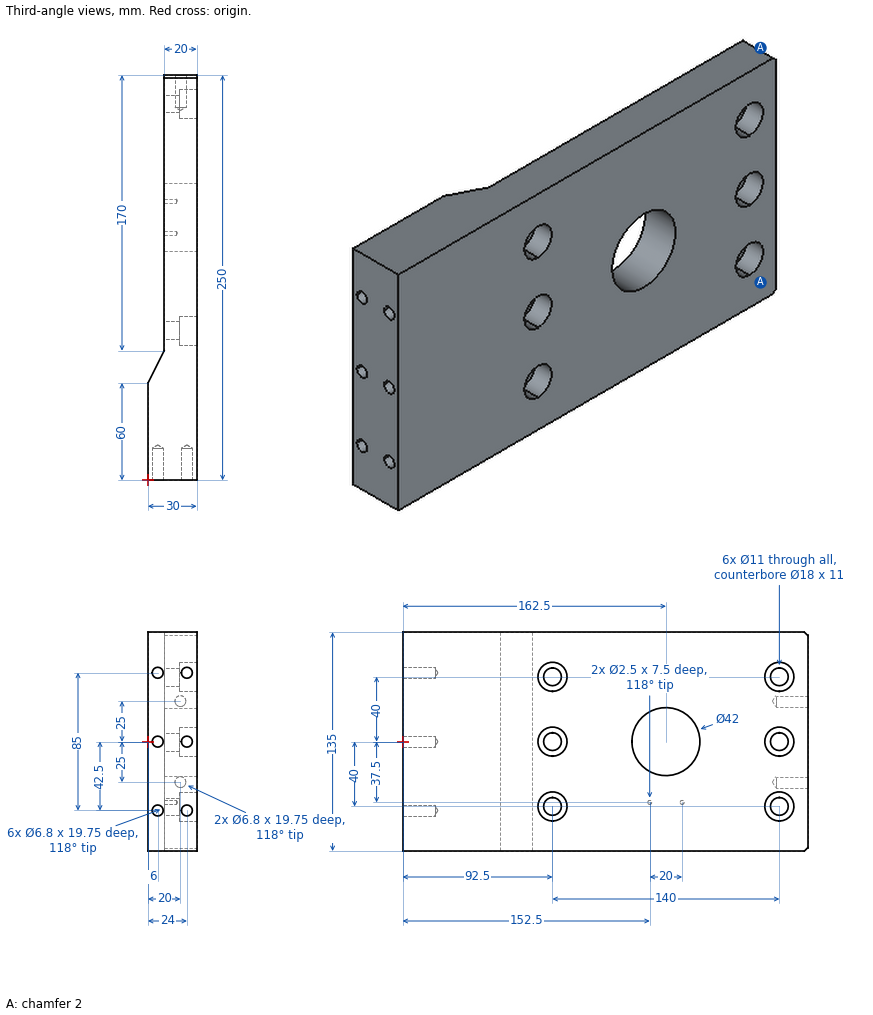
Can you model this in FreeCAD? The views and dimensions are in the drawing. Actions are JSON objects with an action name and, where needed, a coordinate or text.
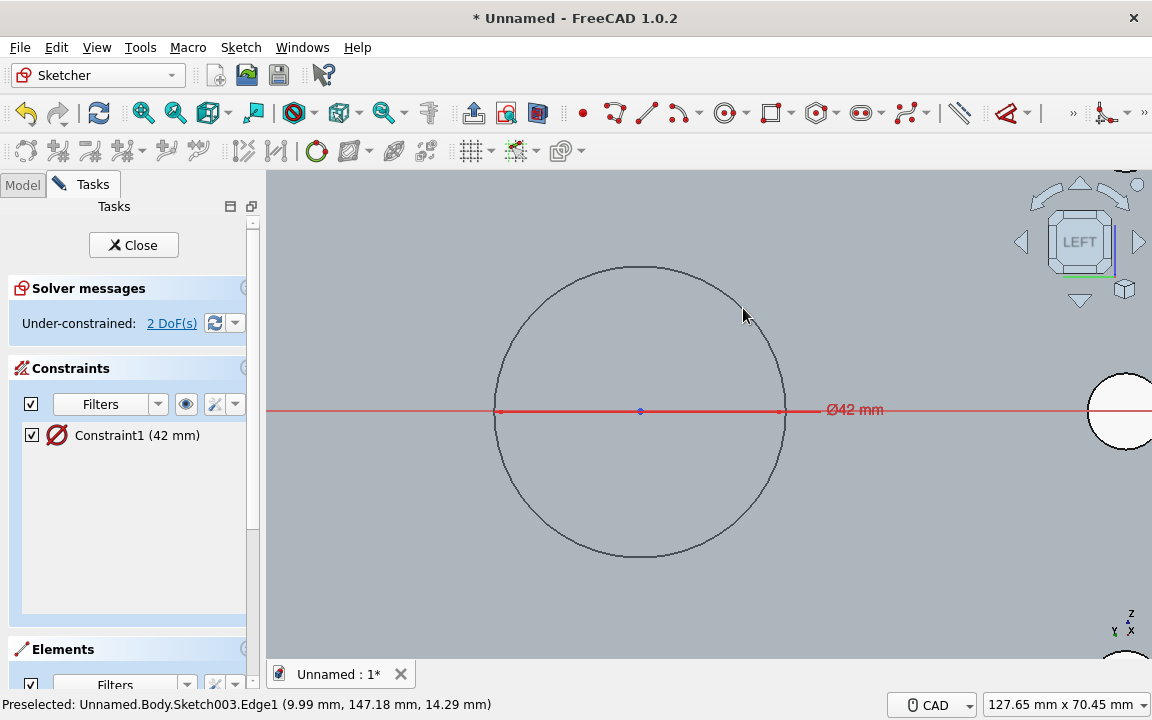
{"action": "left_click", "coordinate": [640, 412]}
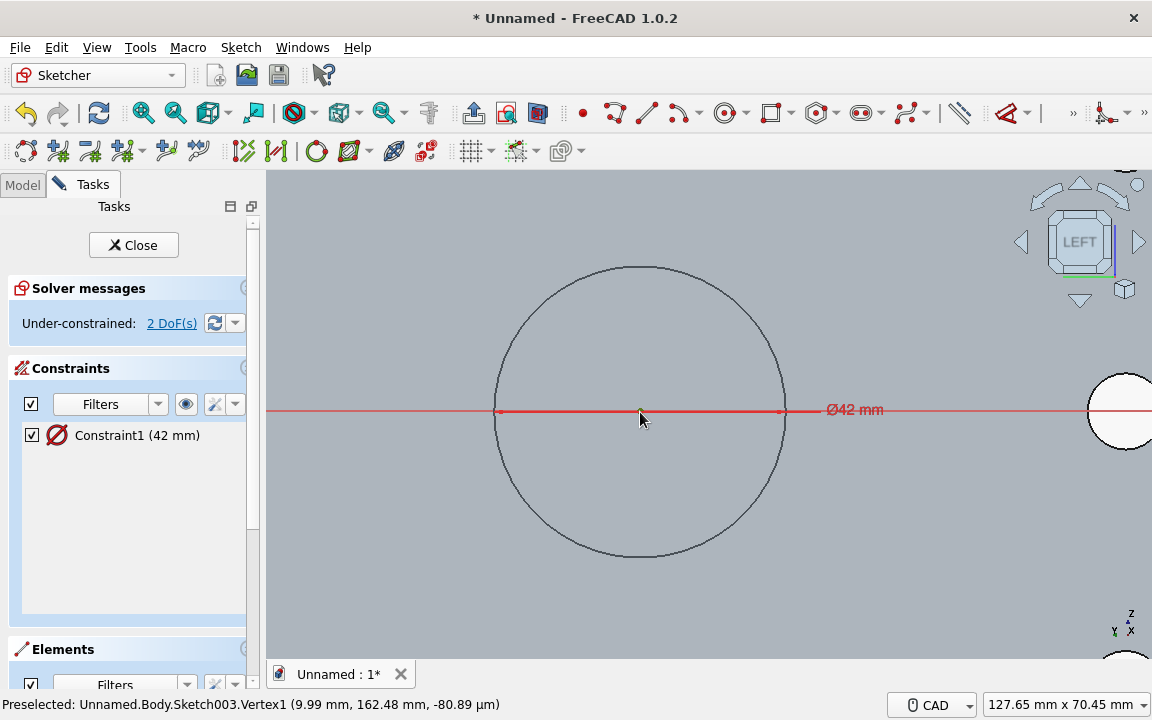
{"action": "left_click", "coordinate": [344, 411]}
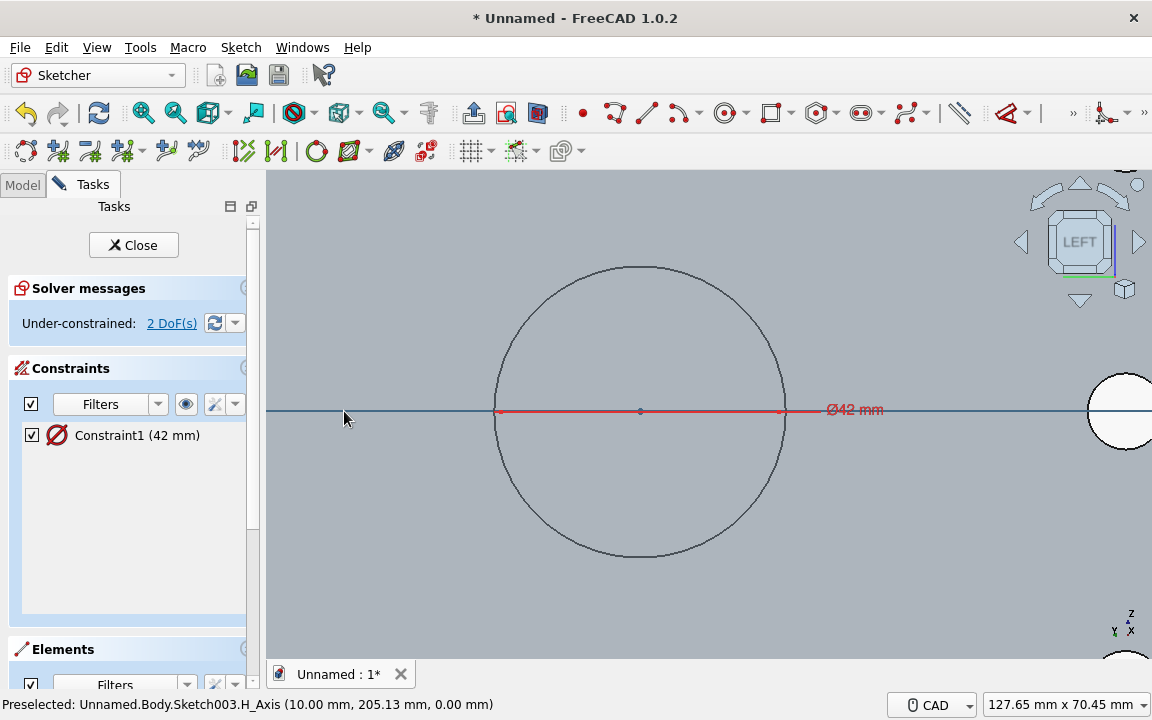
{"action": "key", "text": "c"}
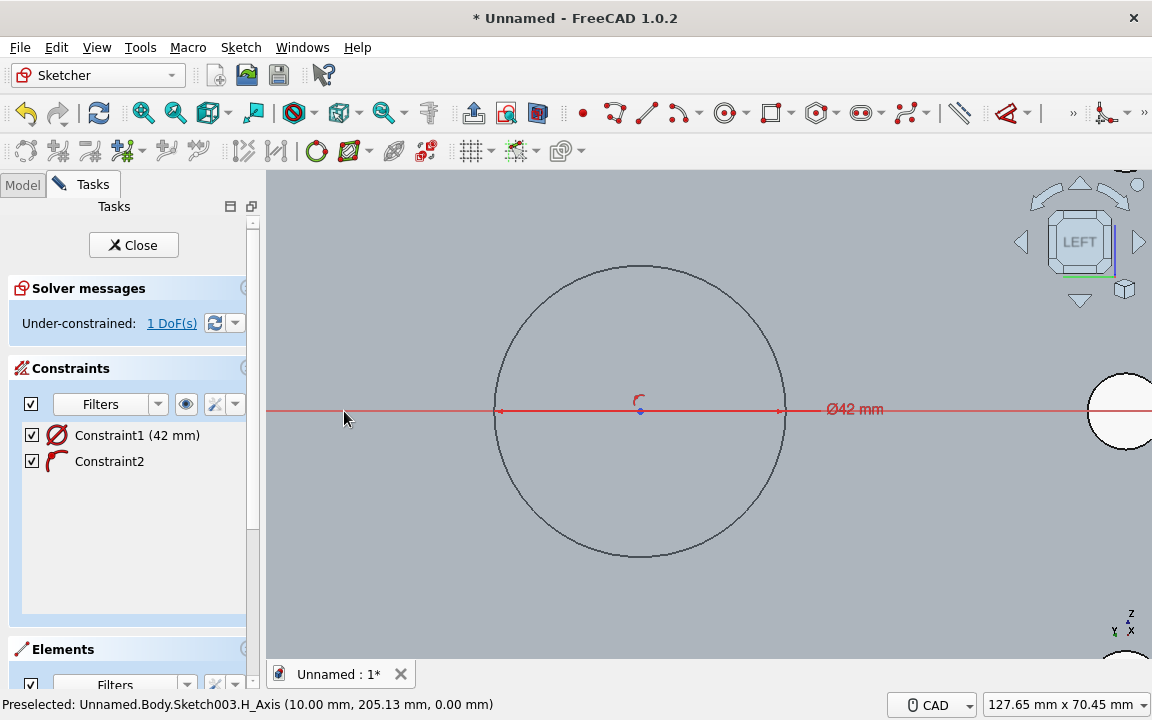
{"action": "left_click", "coordinate": [1006, 114]}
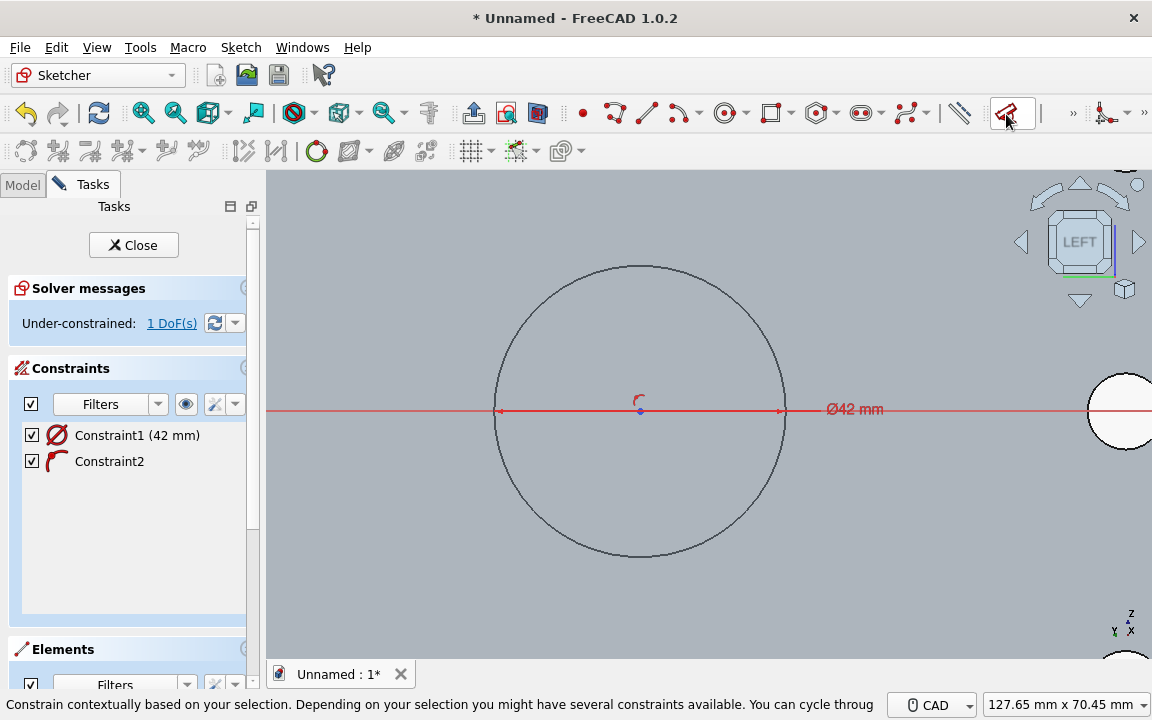
{"action": "left_click", "coordinate": [640, 411]}
{"action": "left_click", "coordinate": [813, 445]}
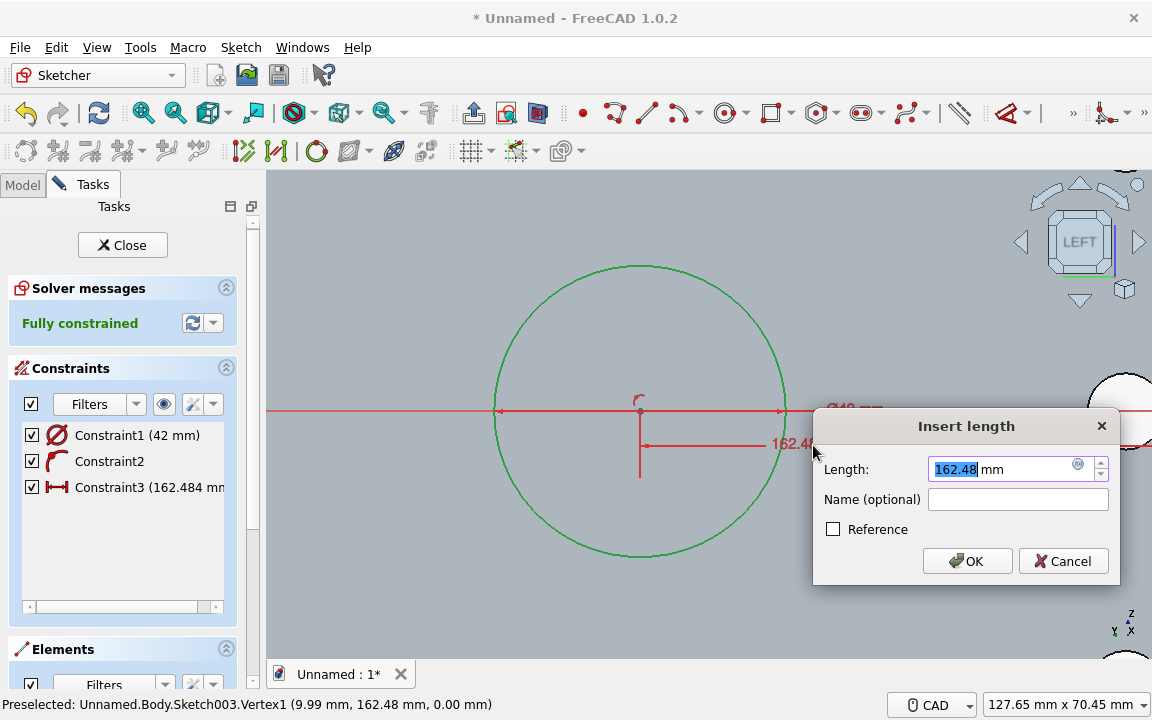
{"action": "type", "text": "162.5"}
{"action": "key", "text": "Return"}
{"action": "key", "text": "Escape"}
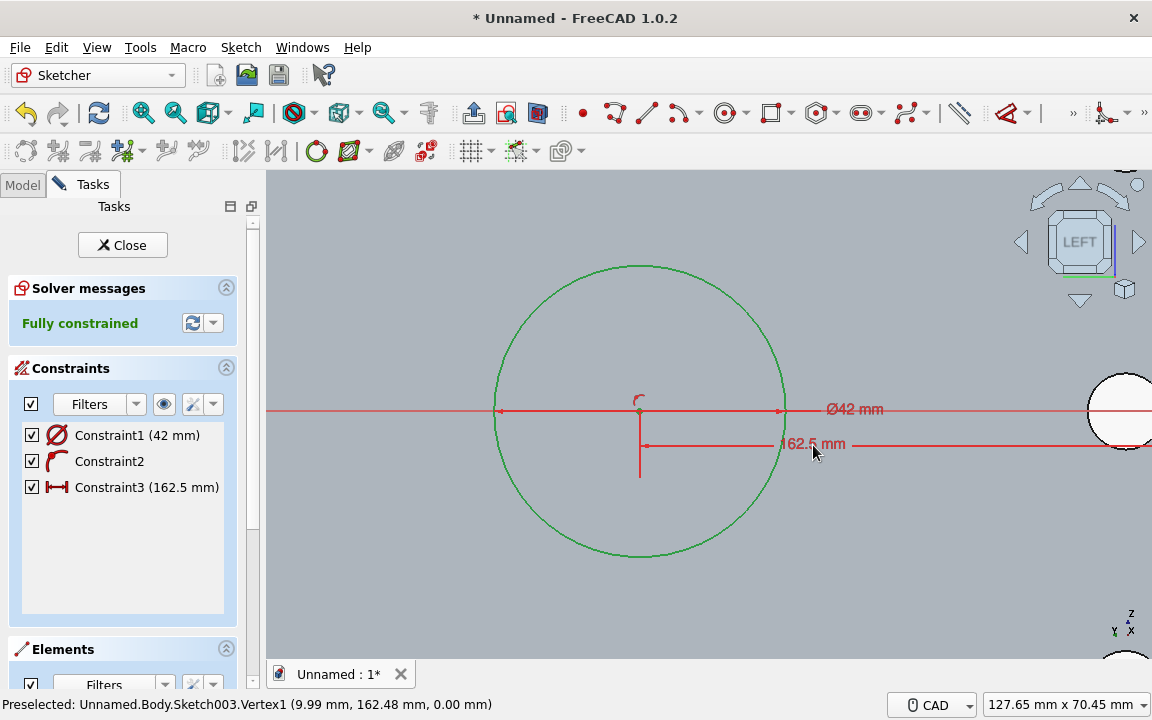
{"action": "left_click", "coordinate": [123, 245]}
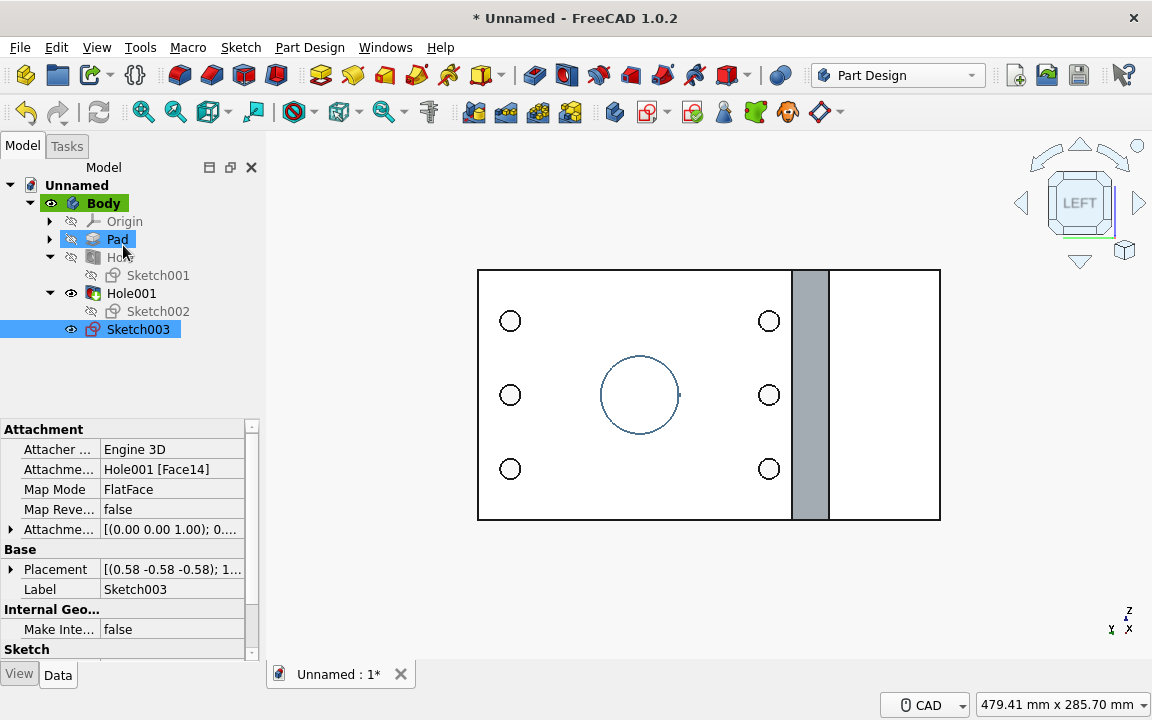
{"action": "left_click", "coordinate": [536, 76]}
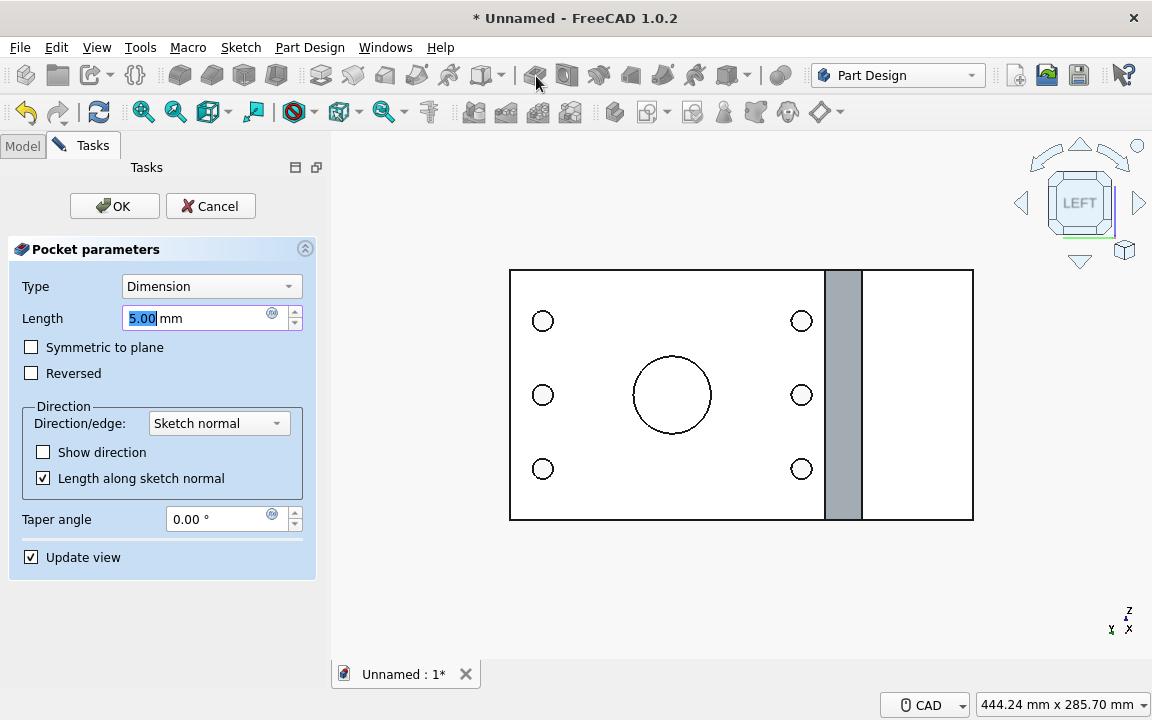
{"action": "left_click", "coordinate": [212, 286]}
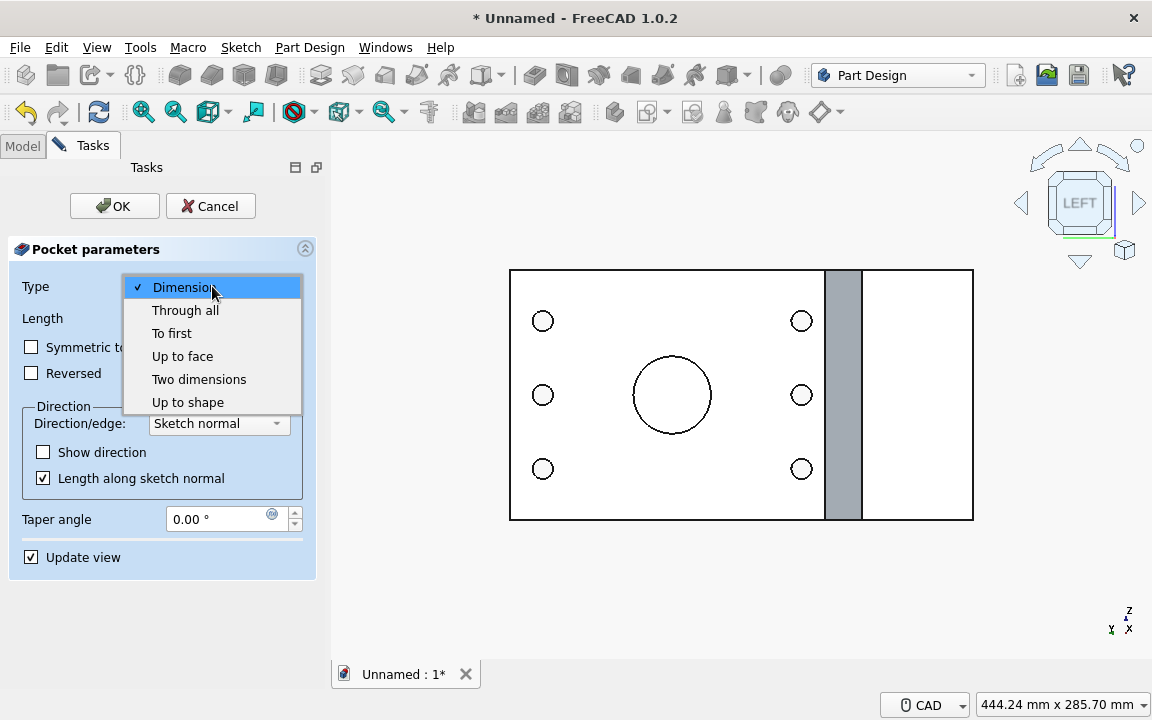
{"action": "left_click", "coordinate": [212, 310]}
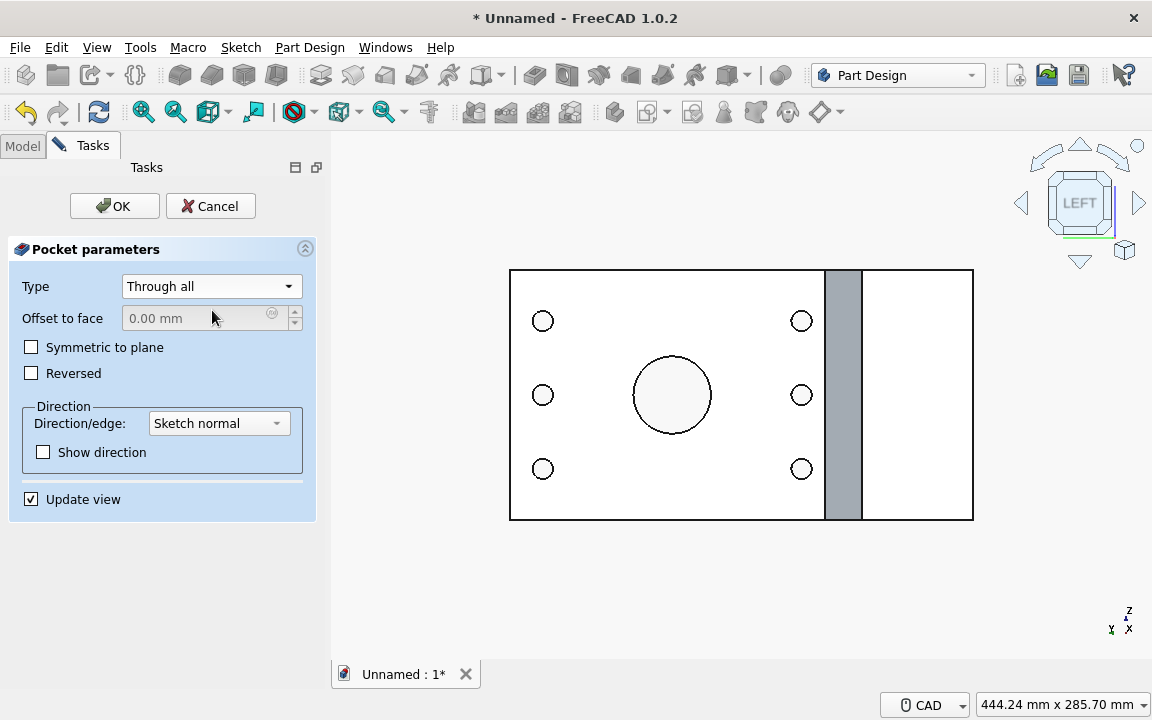
{"action": "left_click", "coordinate": [115, 206]}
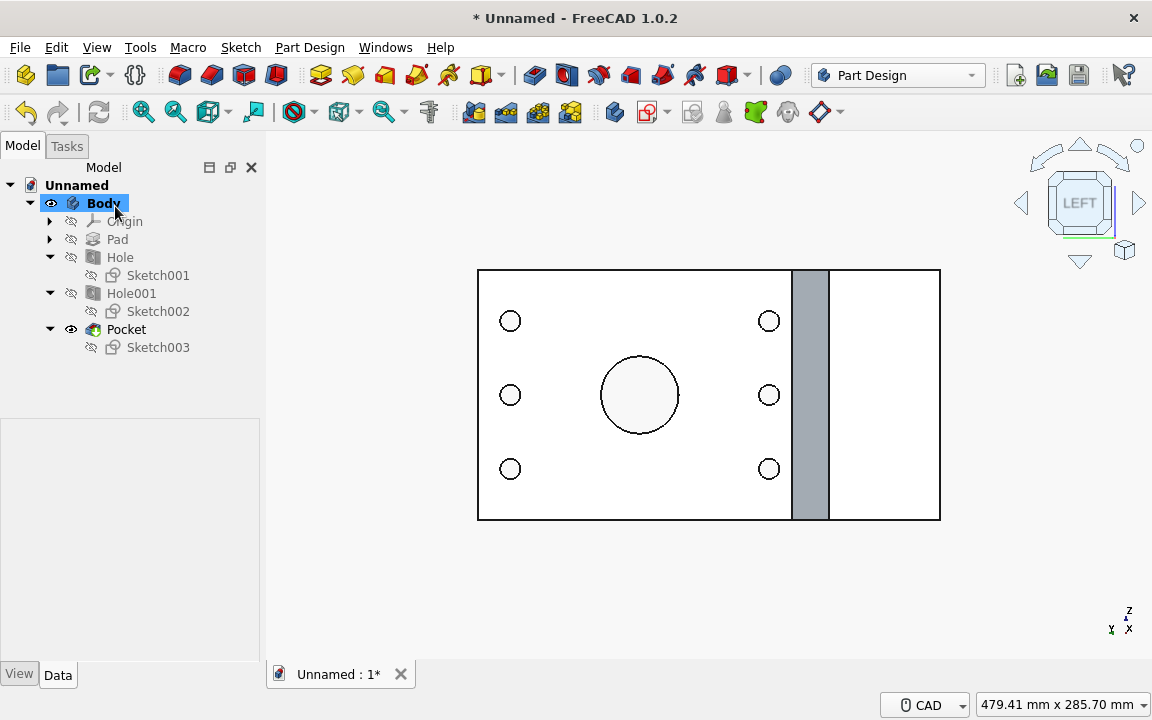
{"action": "key", "text": "4"}